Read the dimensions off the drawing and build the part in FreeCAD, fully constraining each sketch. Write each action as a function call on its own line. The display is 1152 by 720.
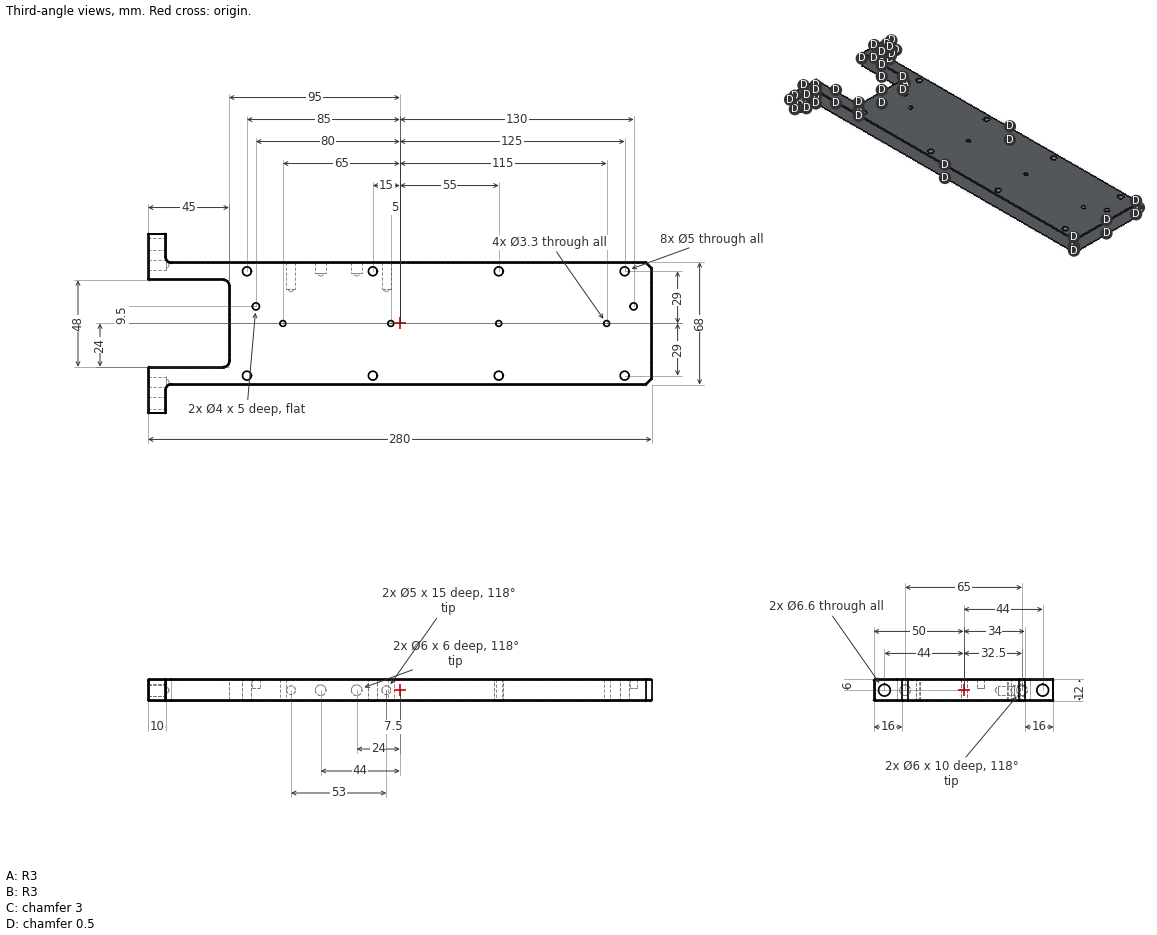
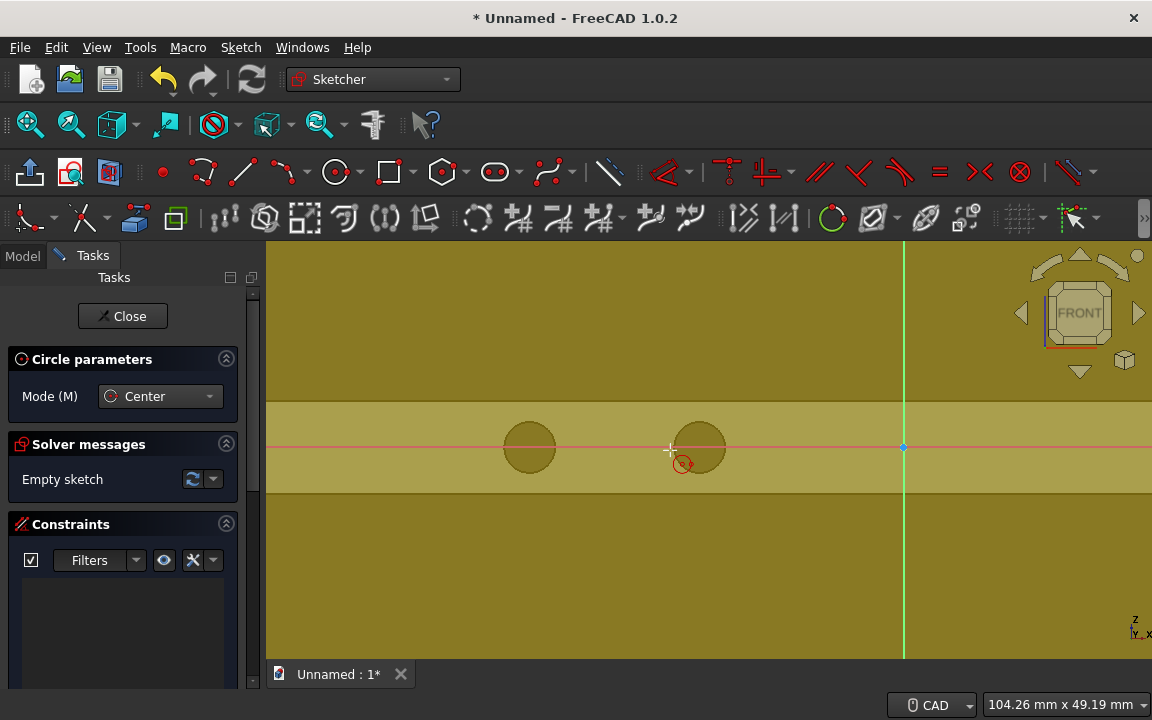
click(840, 447)
move(855, 432)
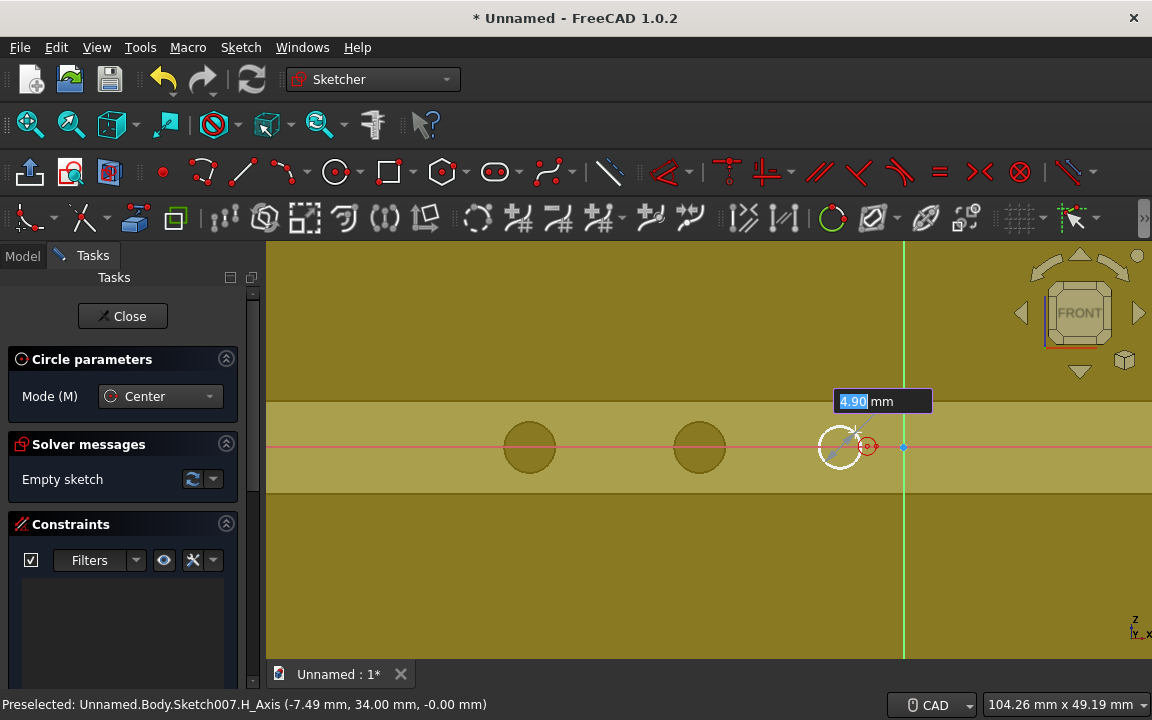
text(5)
key(Return)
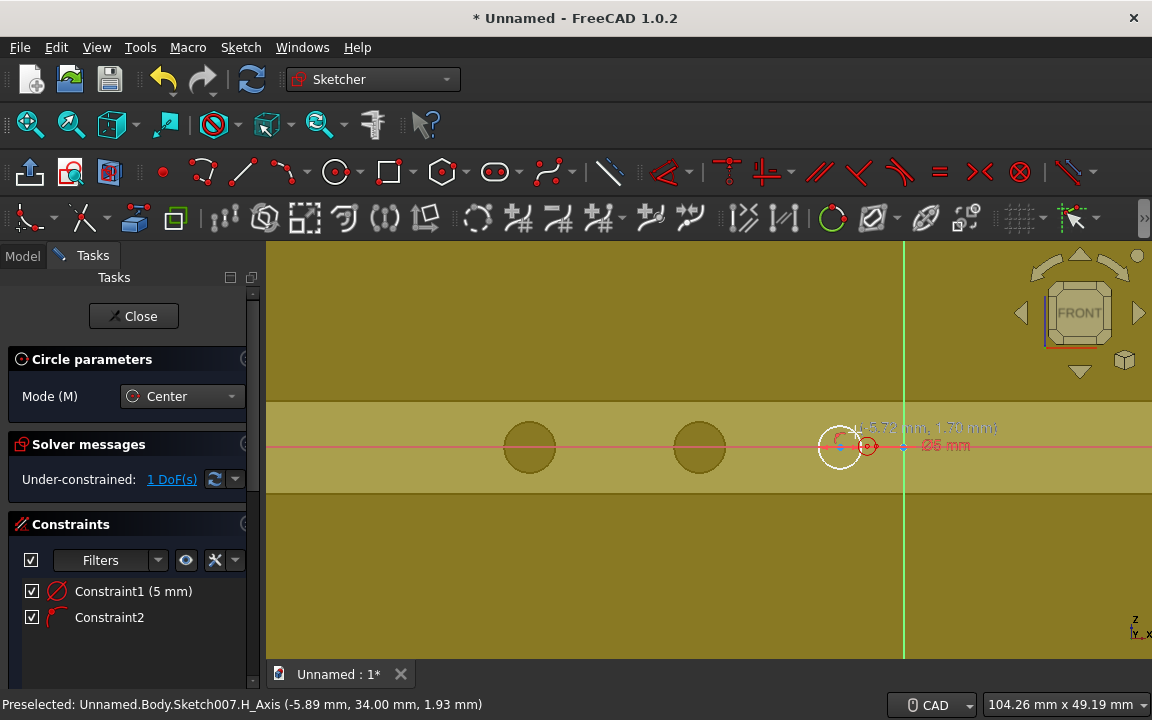
click(389, 447)
move(405, 432)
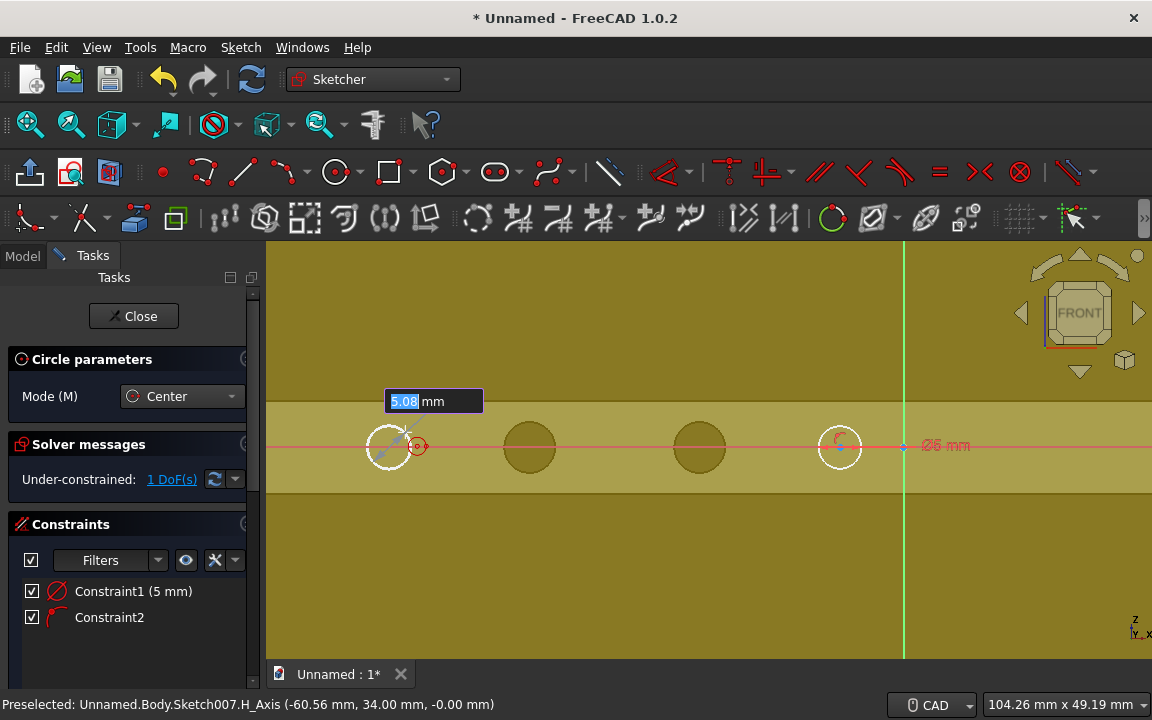
text(5)
key(Return)
key(Escape)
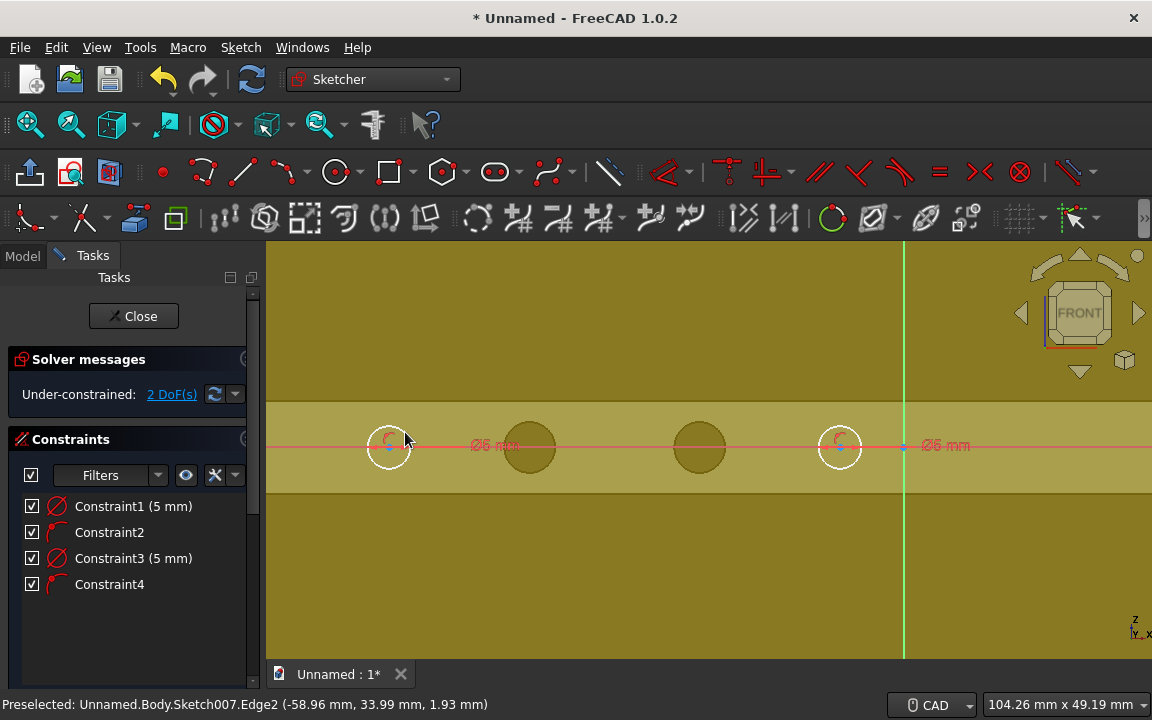
key(d)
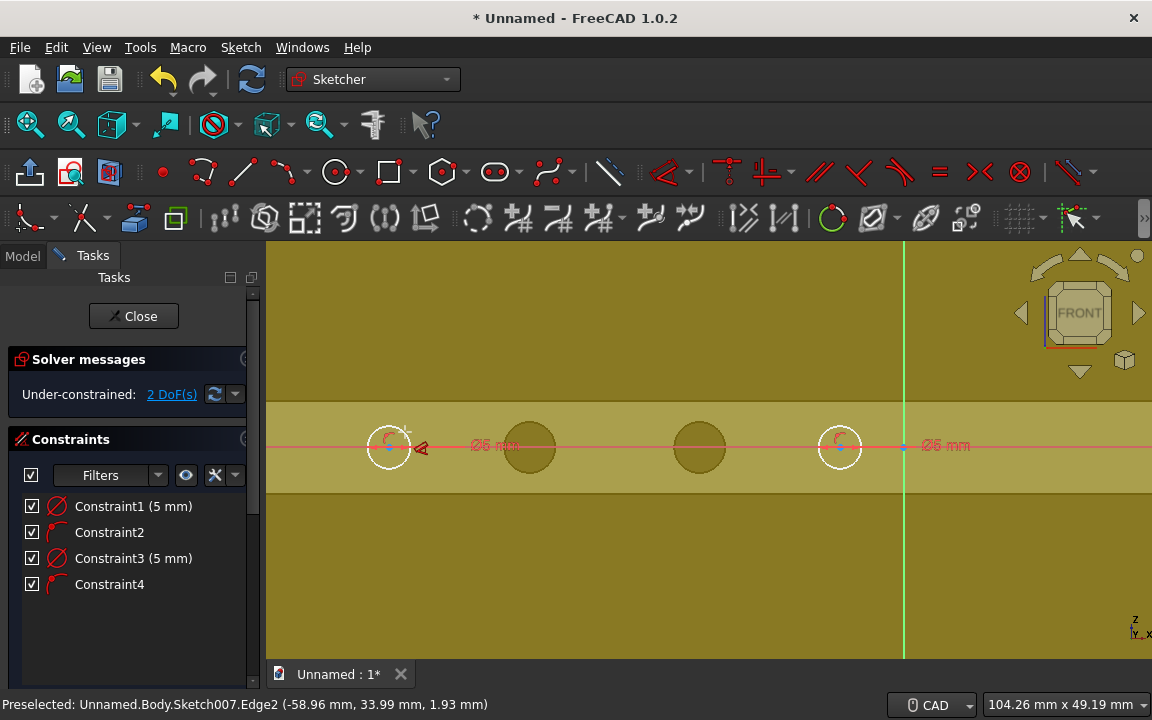
click(840, 447)
click(872, 481)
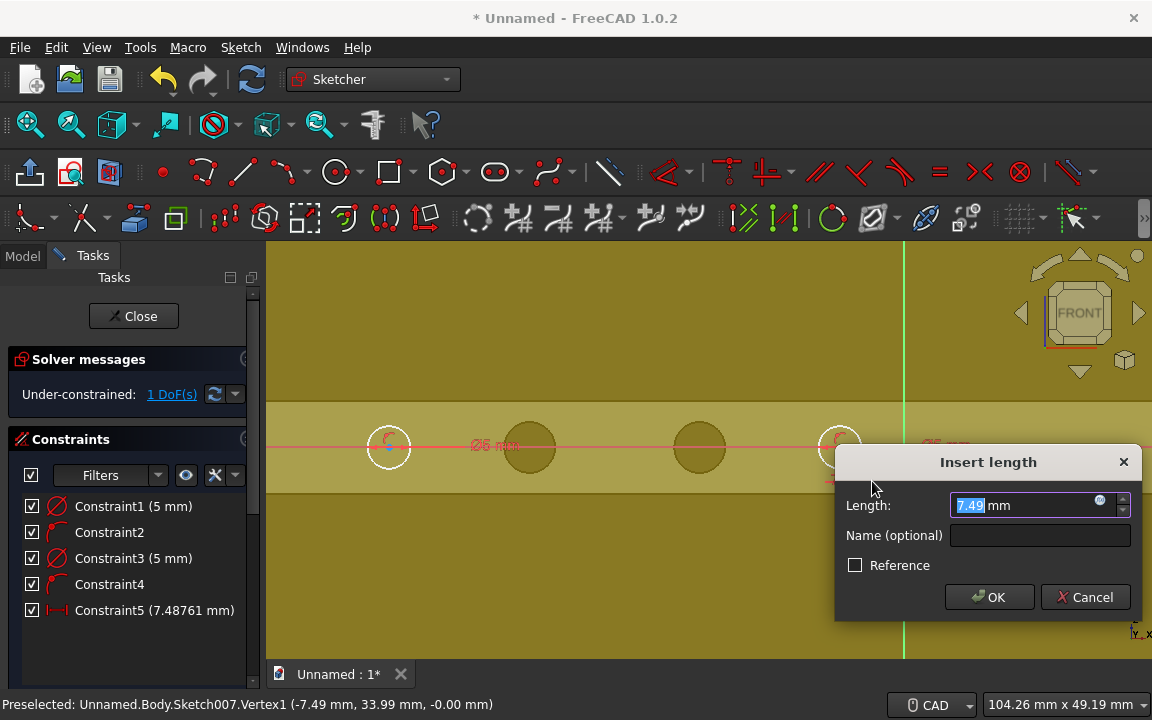
text(7.5)
key(Return)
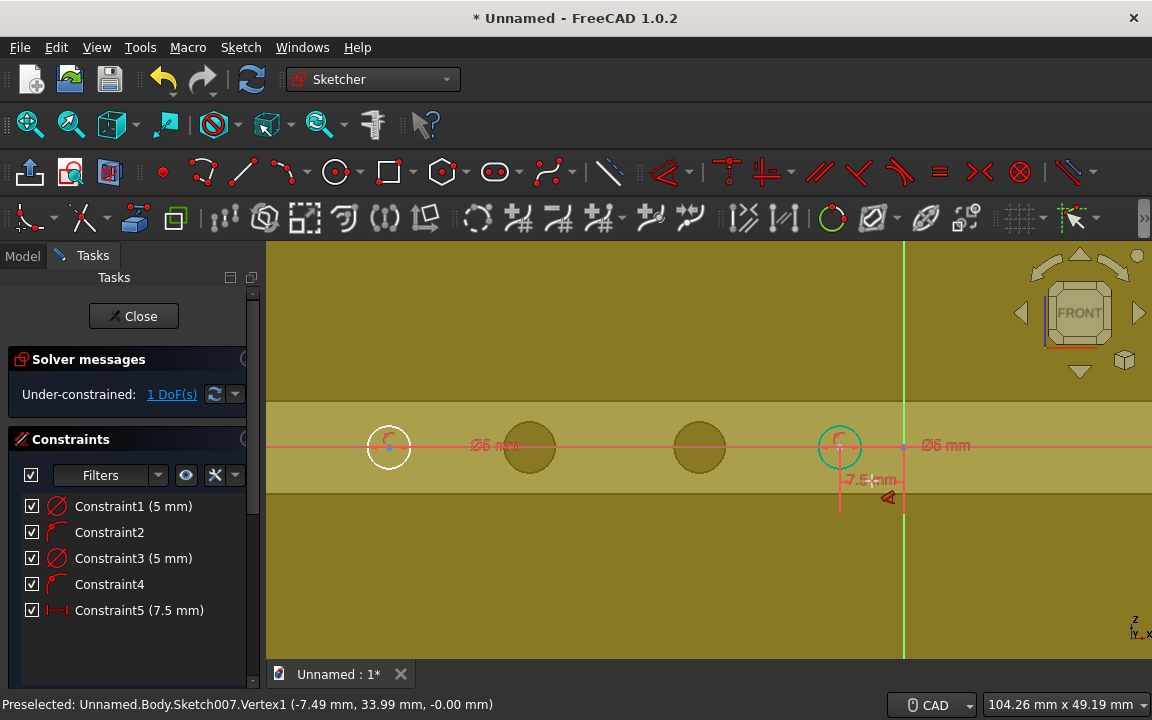
click(840, 447)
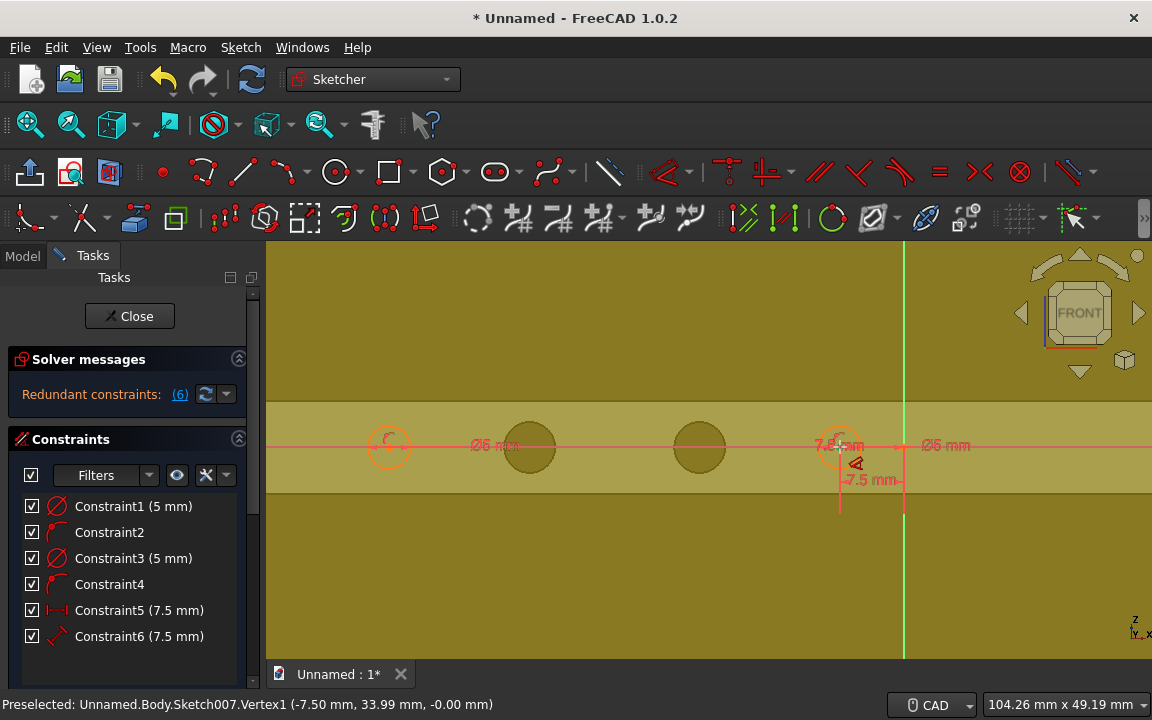
click(389, 447)
click(614, 481)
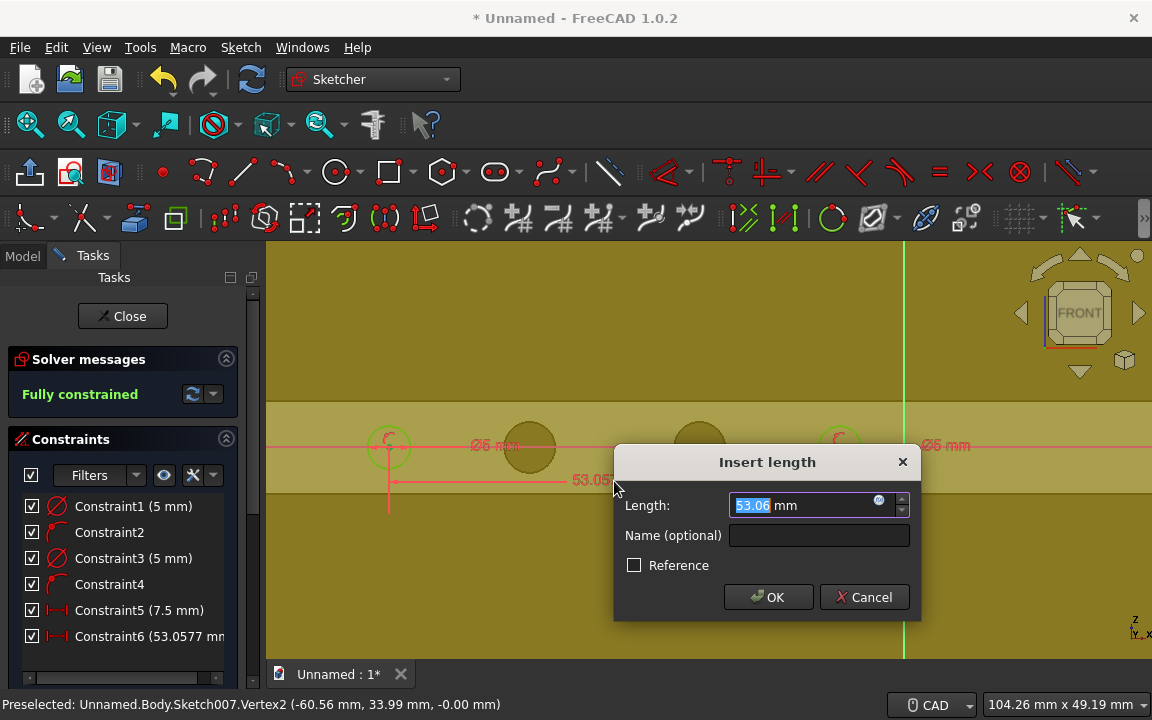
text(53)
key(Return)
key(Escape)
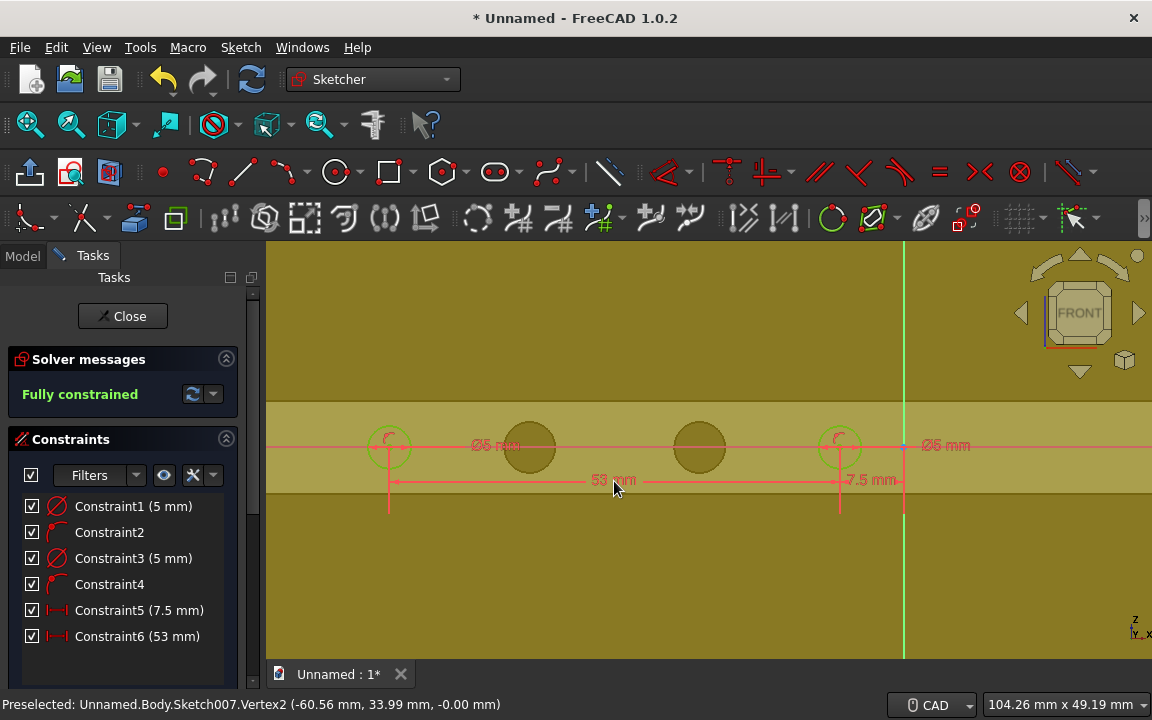
click(123, 316)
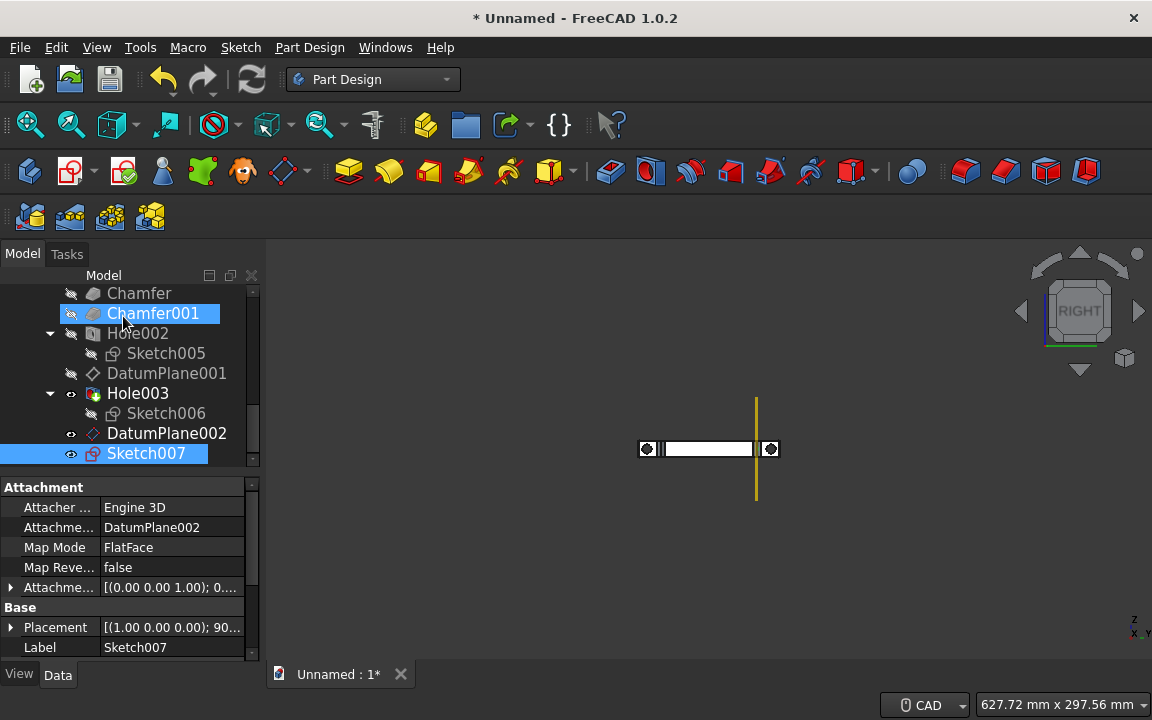
click(652, 172)